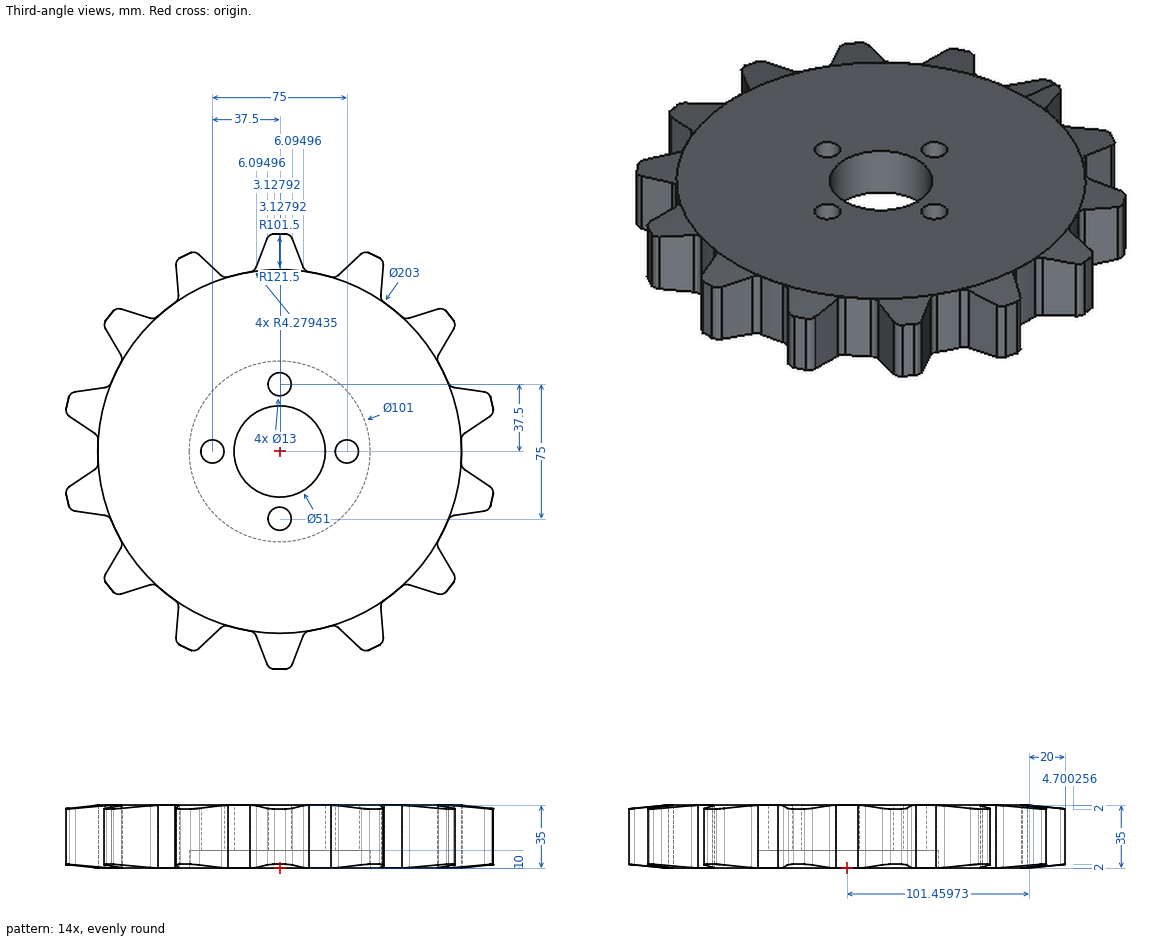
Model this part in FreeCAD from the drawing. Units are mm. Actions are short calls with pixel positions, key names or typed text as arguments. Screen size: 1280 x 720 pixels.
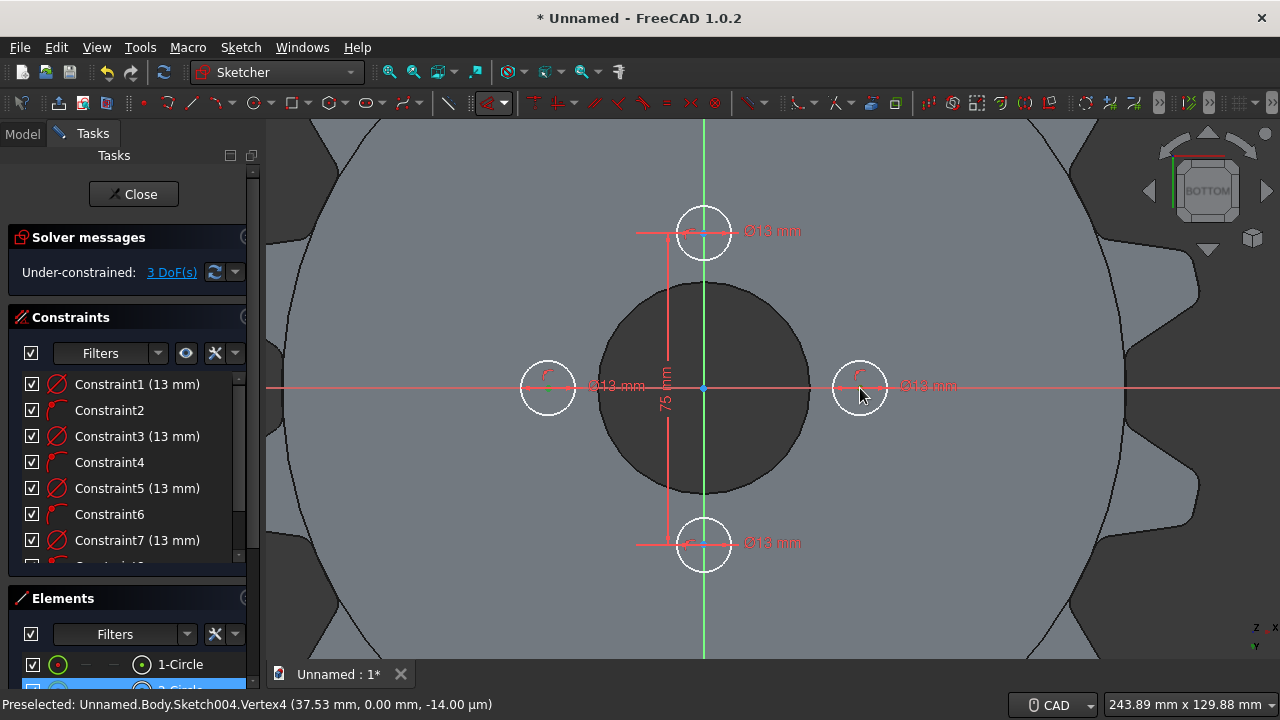
click(506, 104)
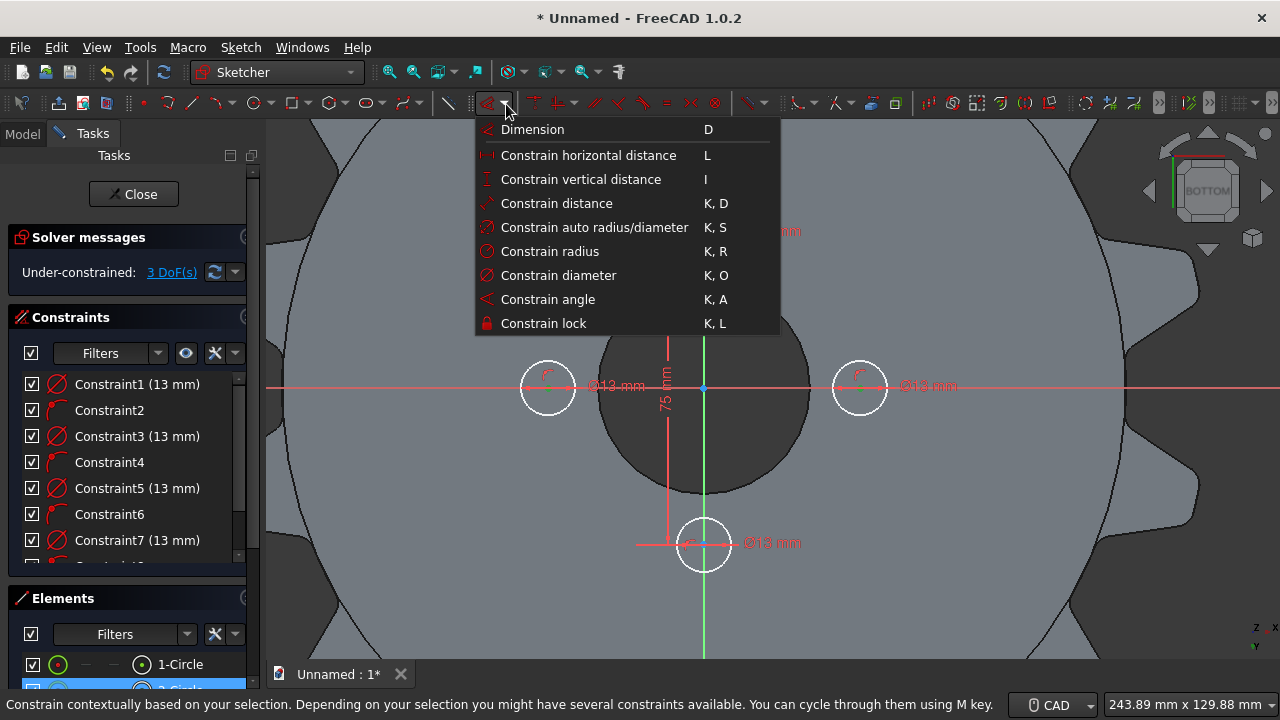
click(628, 155)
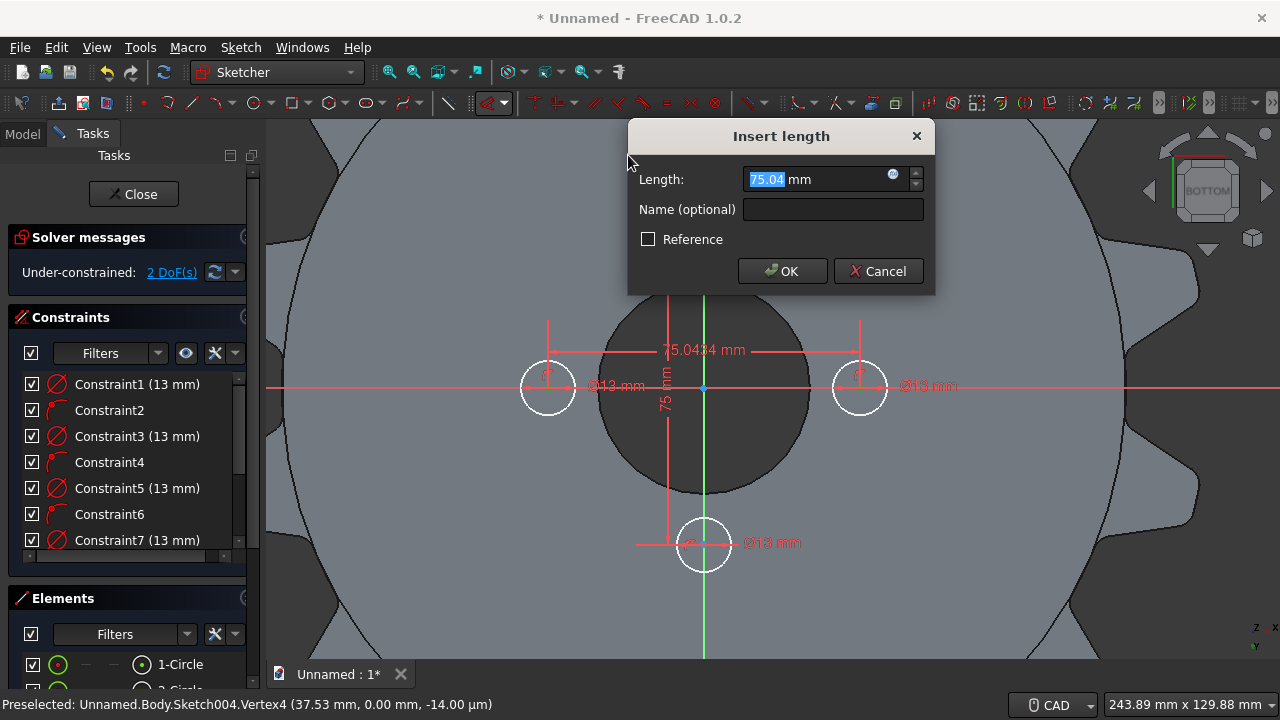
text(75)
key(Return)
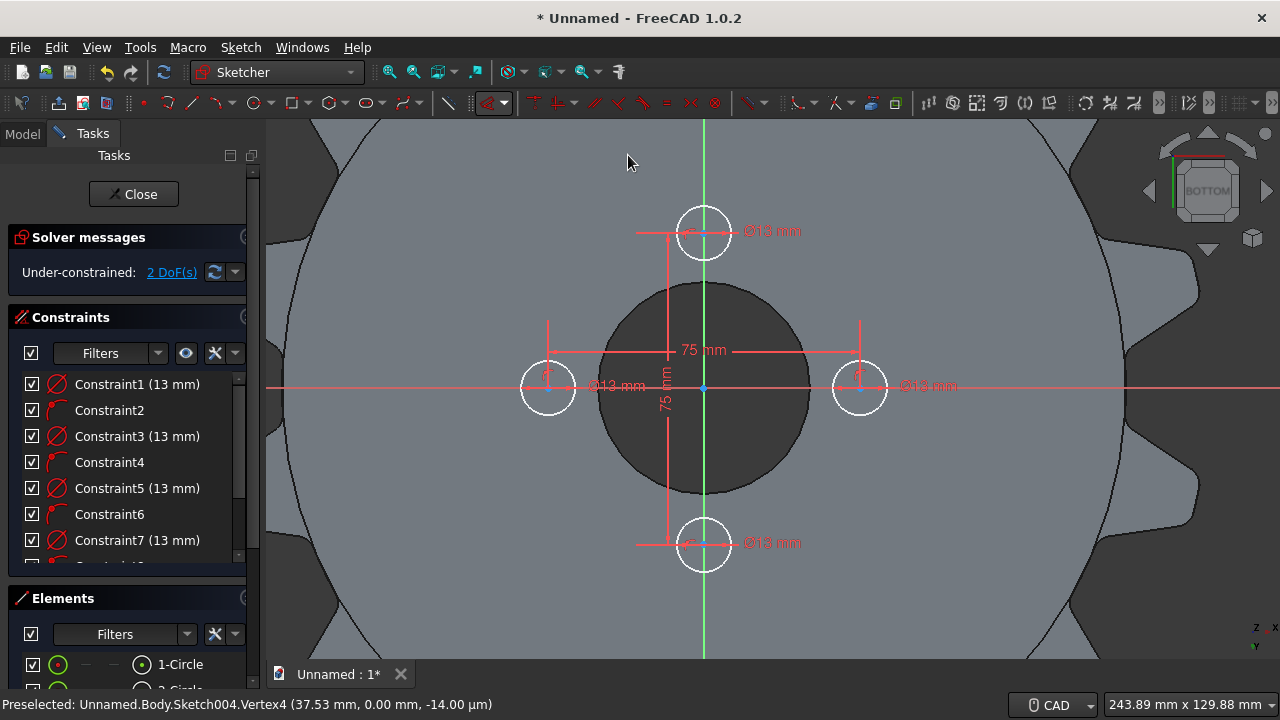
click(704, 545)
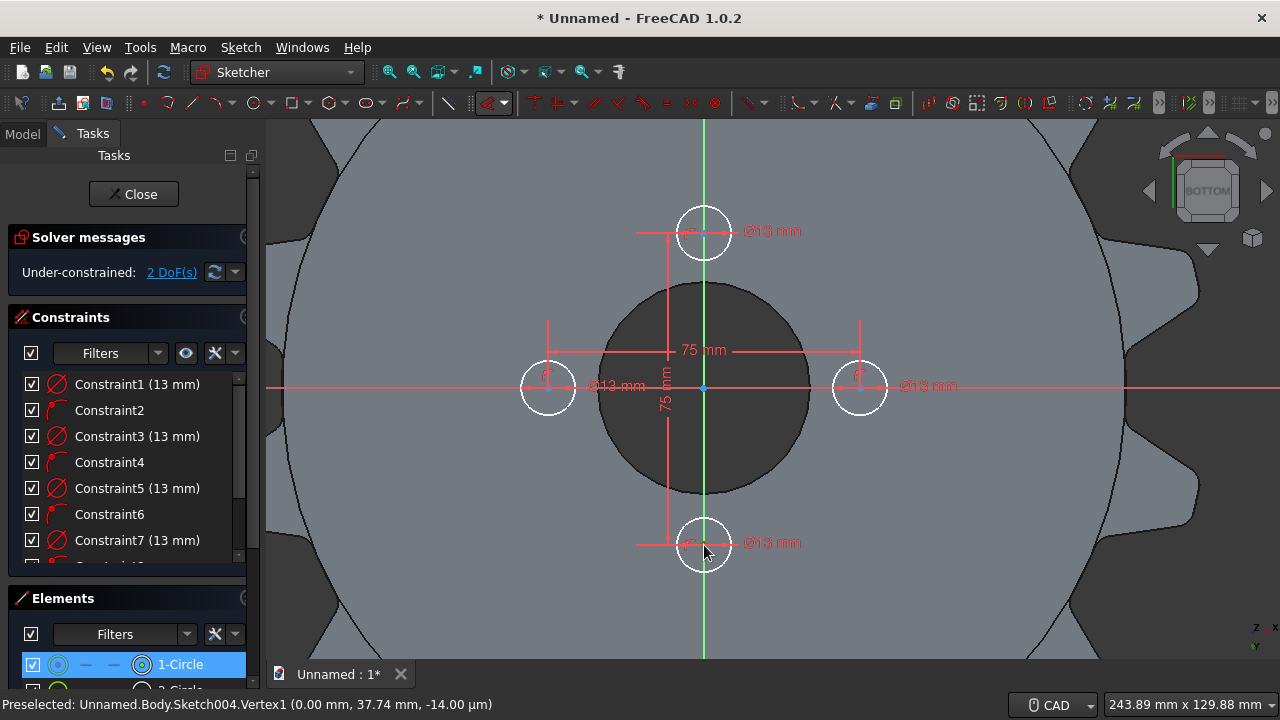
click(506, 104)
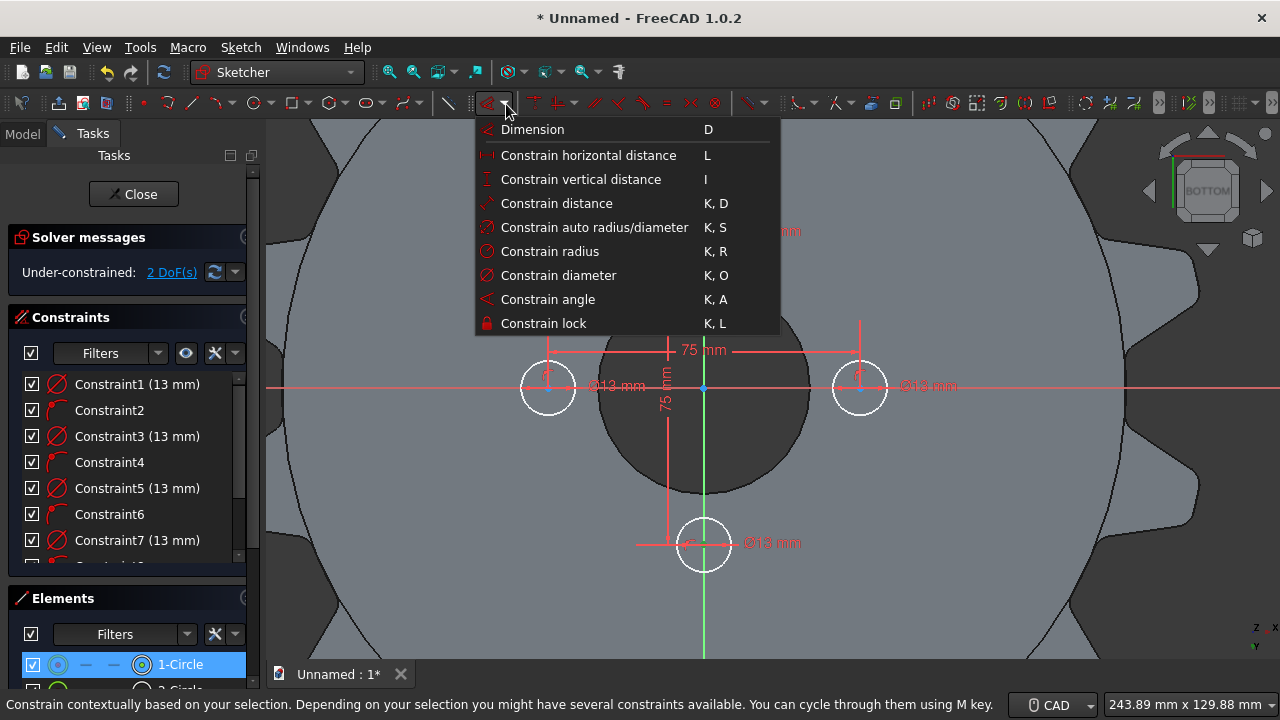
click(628, 179)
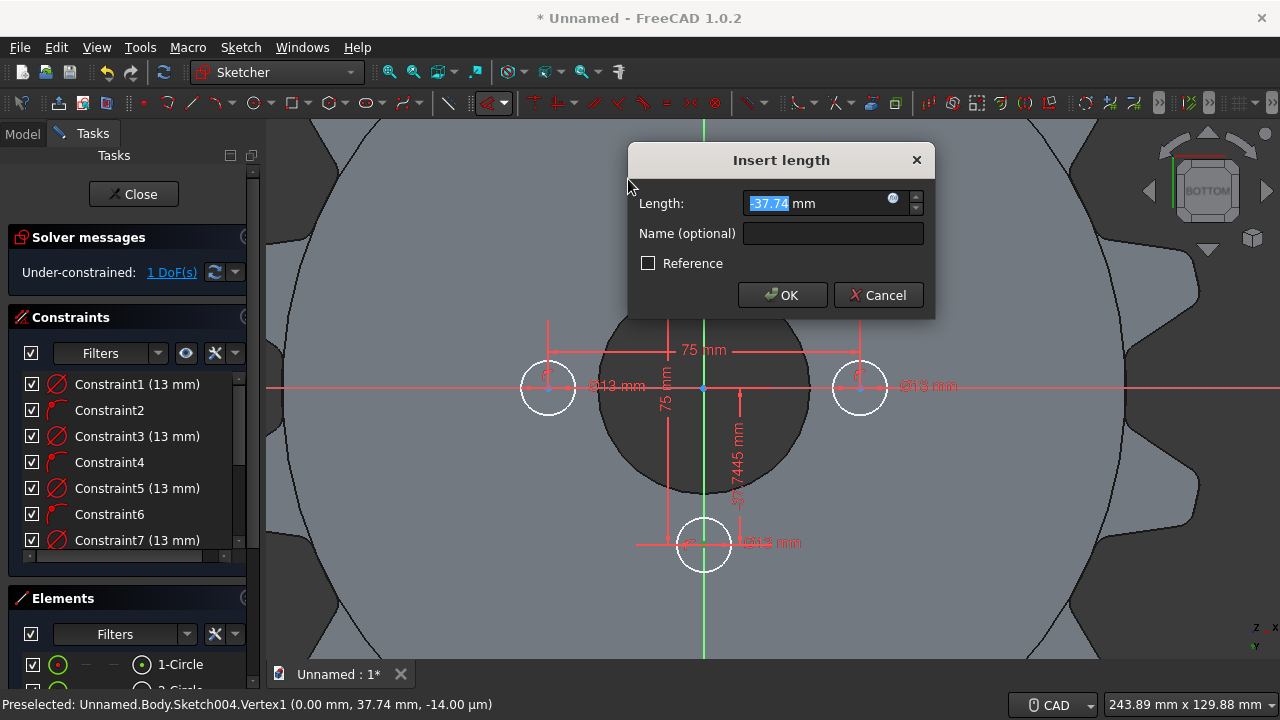
text(-37.5)
key(Return)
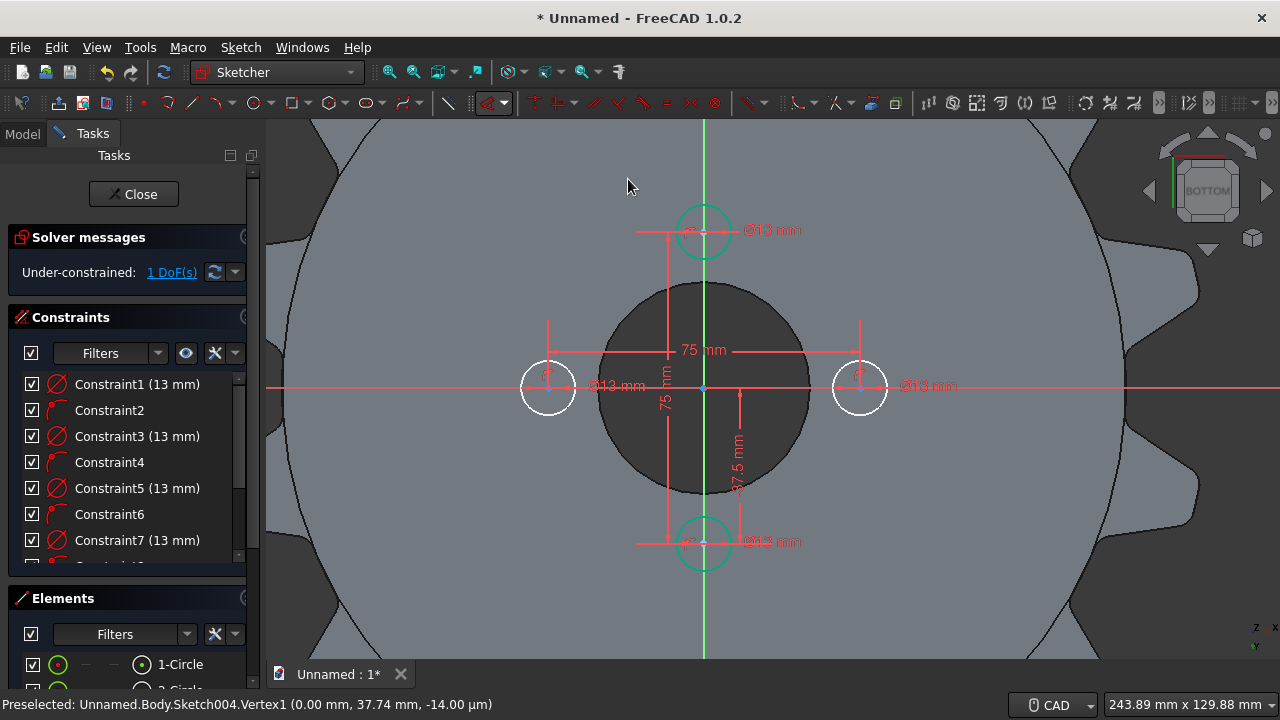
click(548, 388)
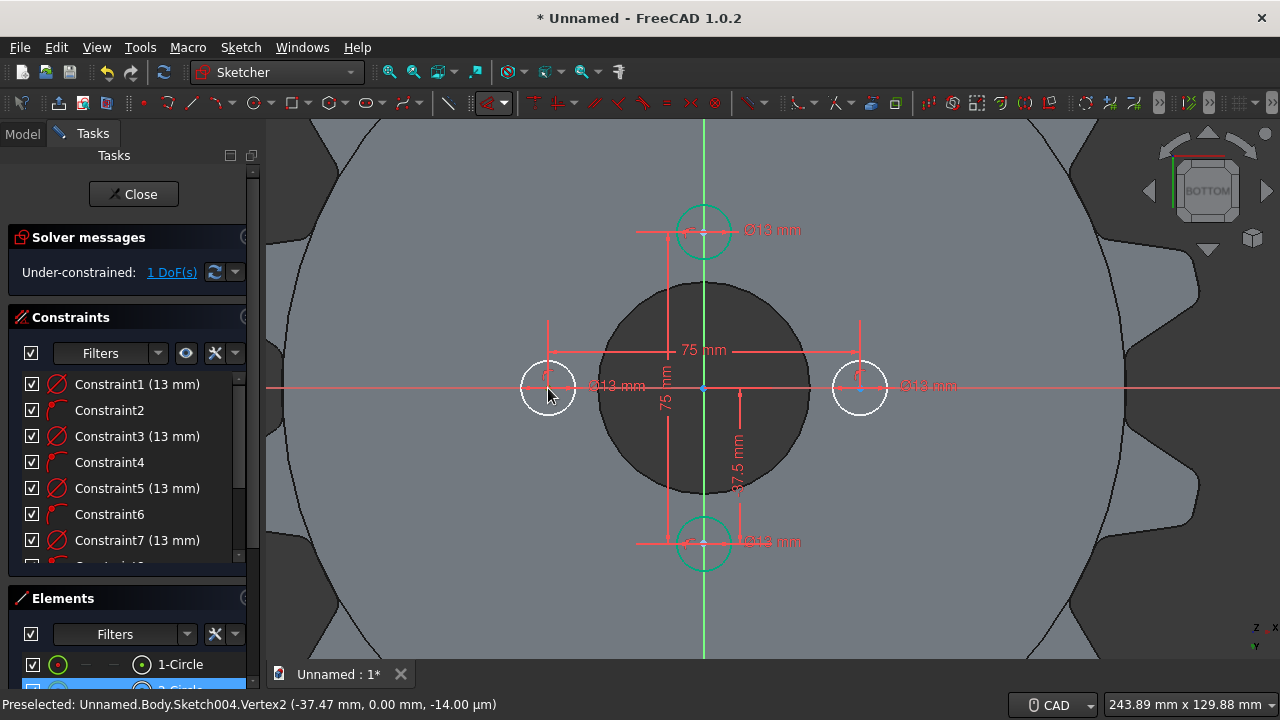
click(506, 104)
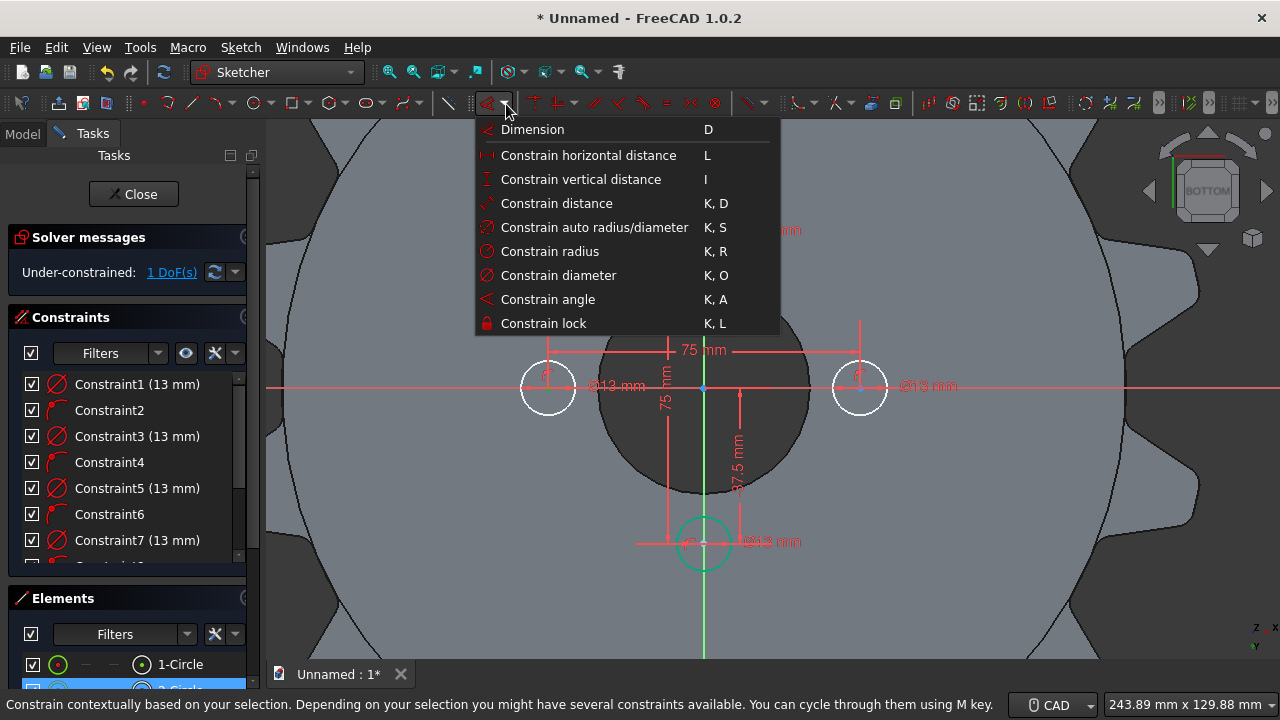
click(628, 155)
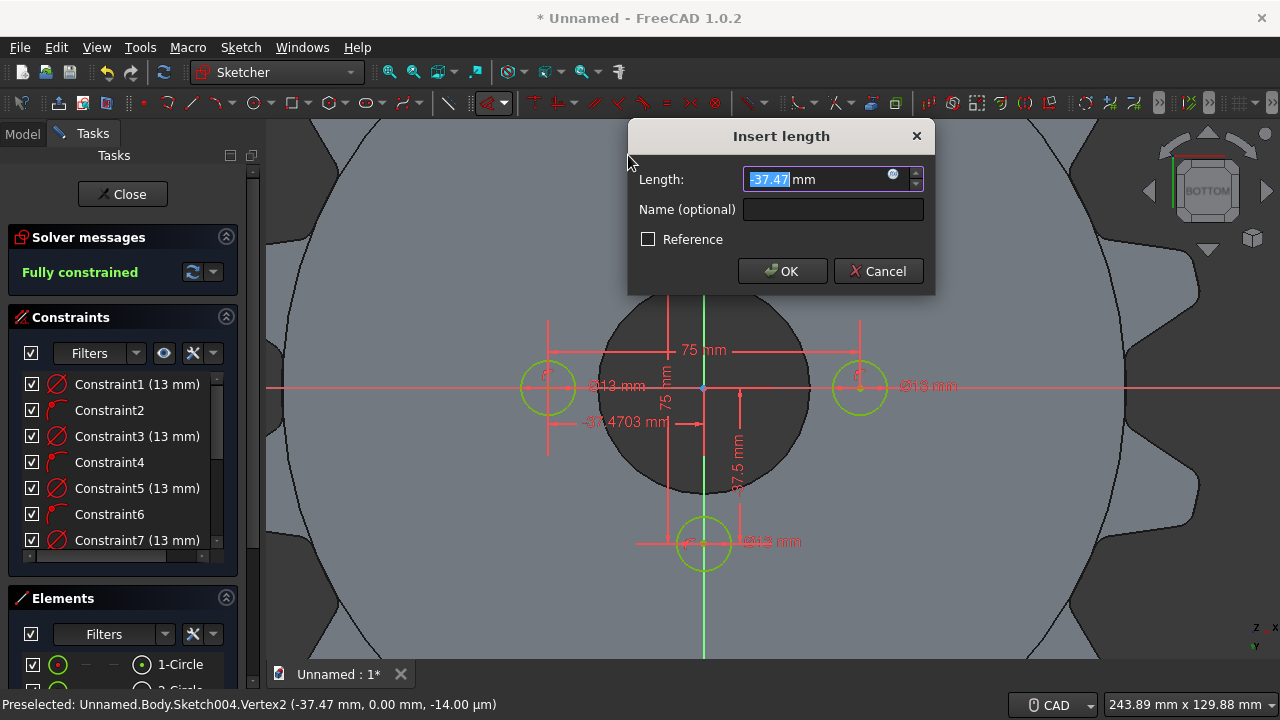
text(-37.5)
key(Return)